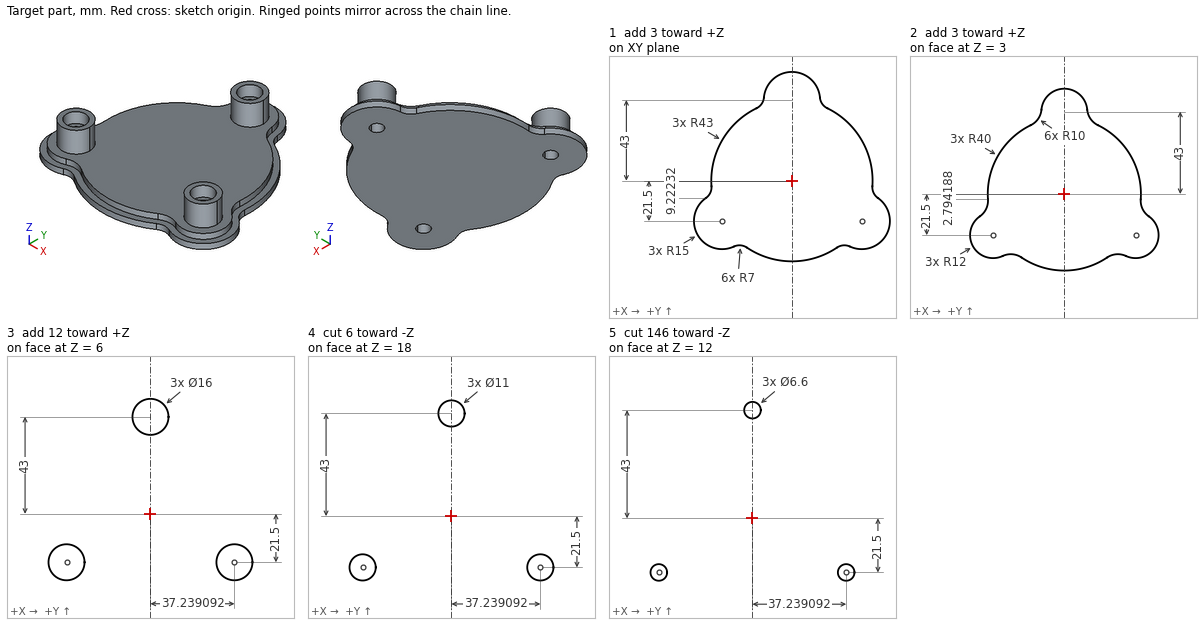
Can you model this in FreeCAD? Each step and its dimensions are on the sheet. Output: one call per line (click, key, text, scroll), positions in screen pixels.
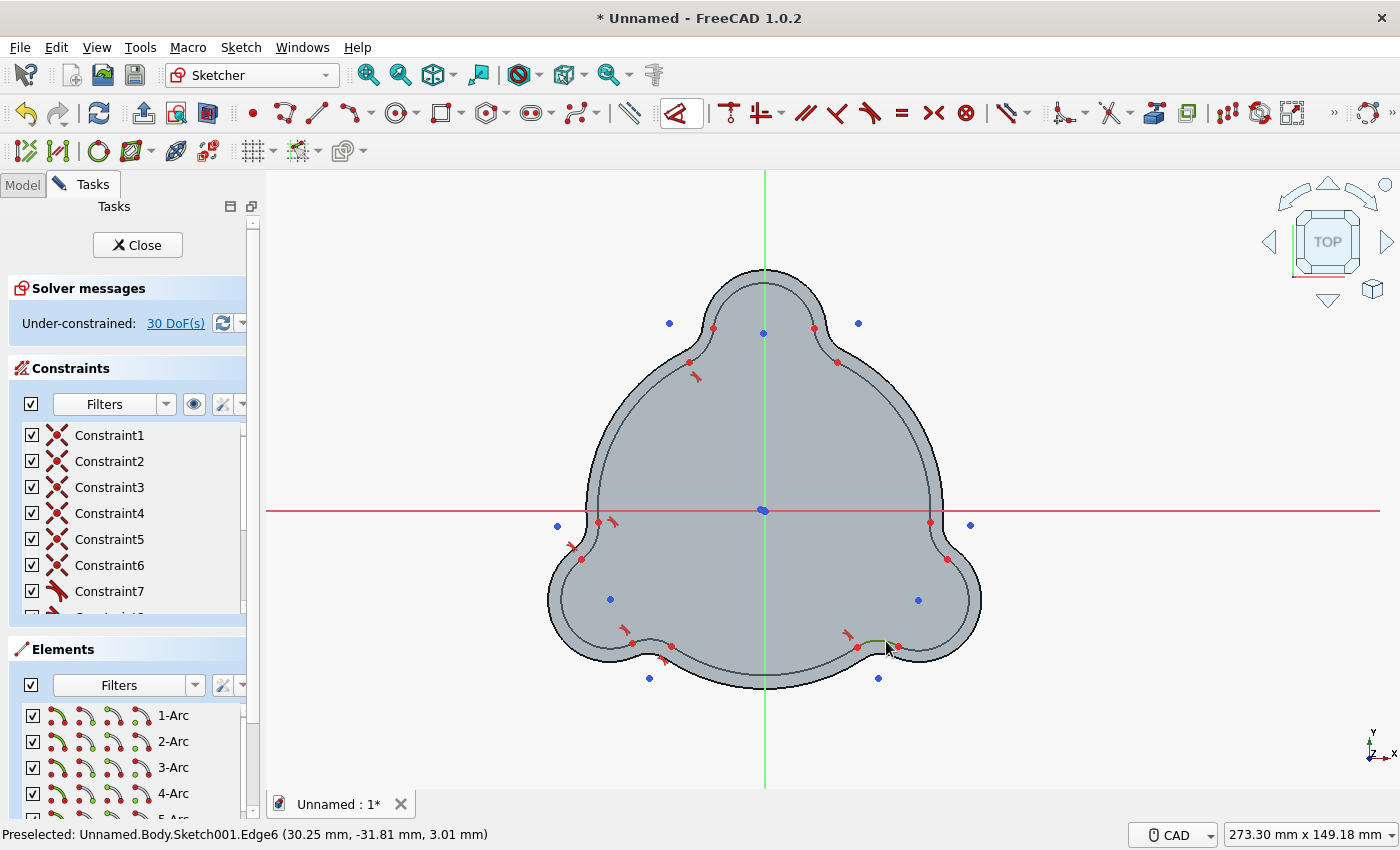
click(941, 645)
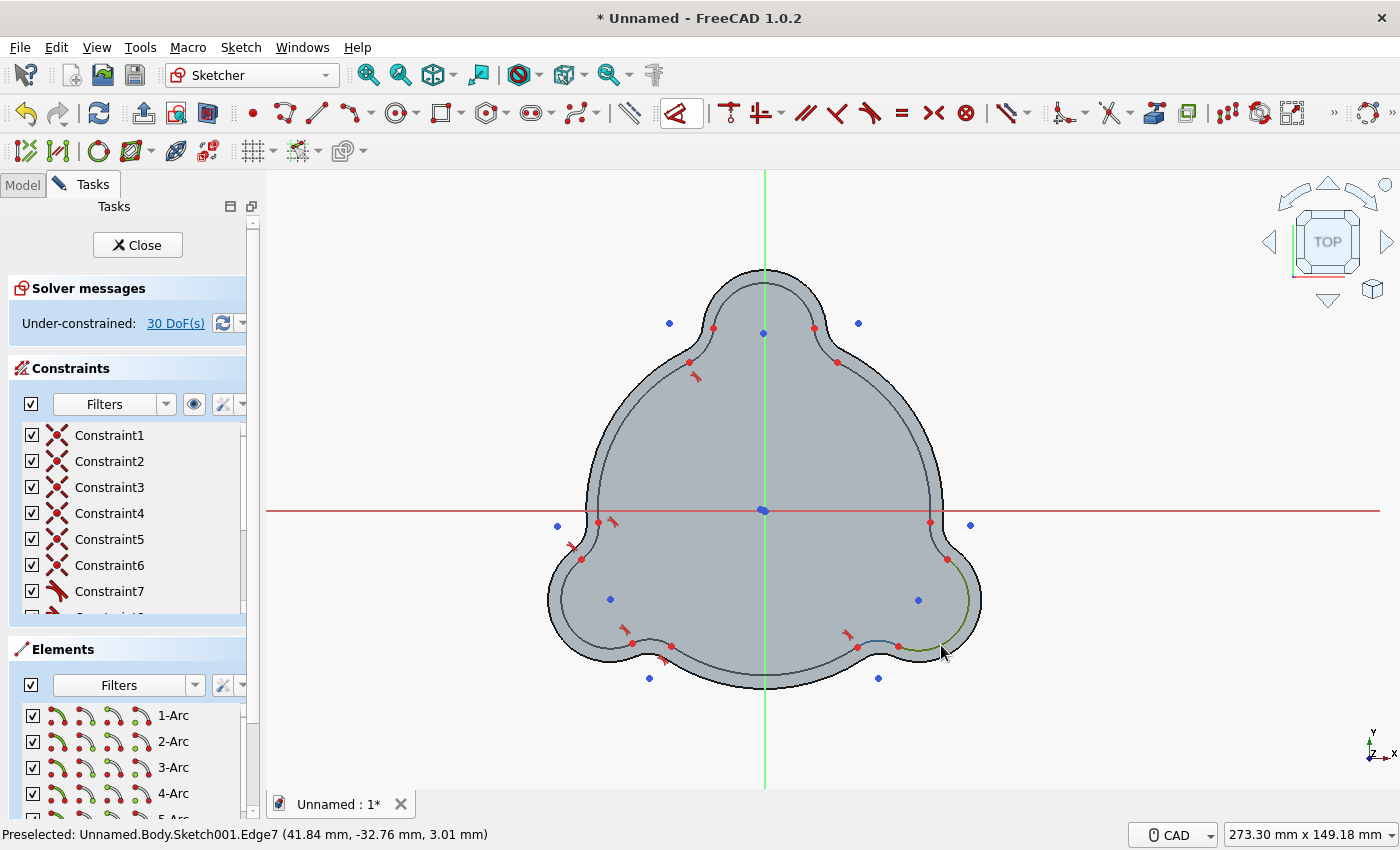
key(t)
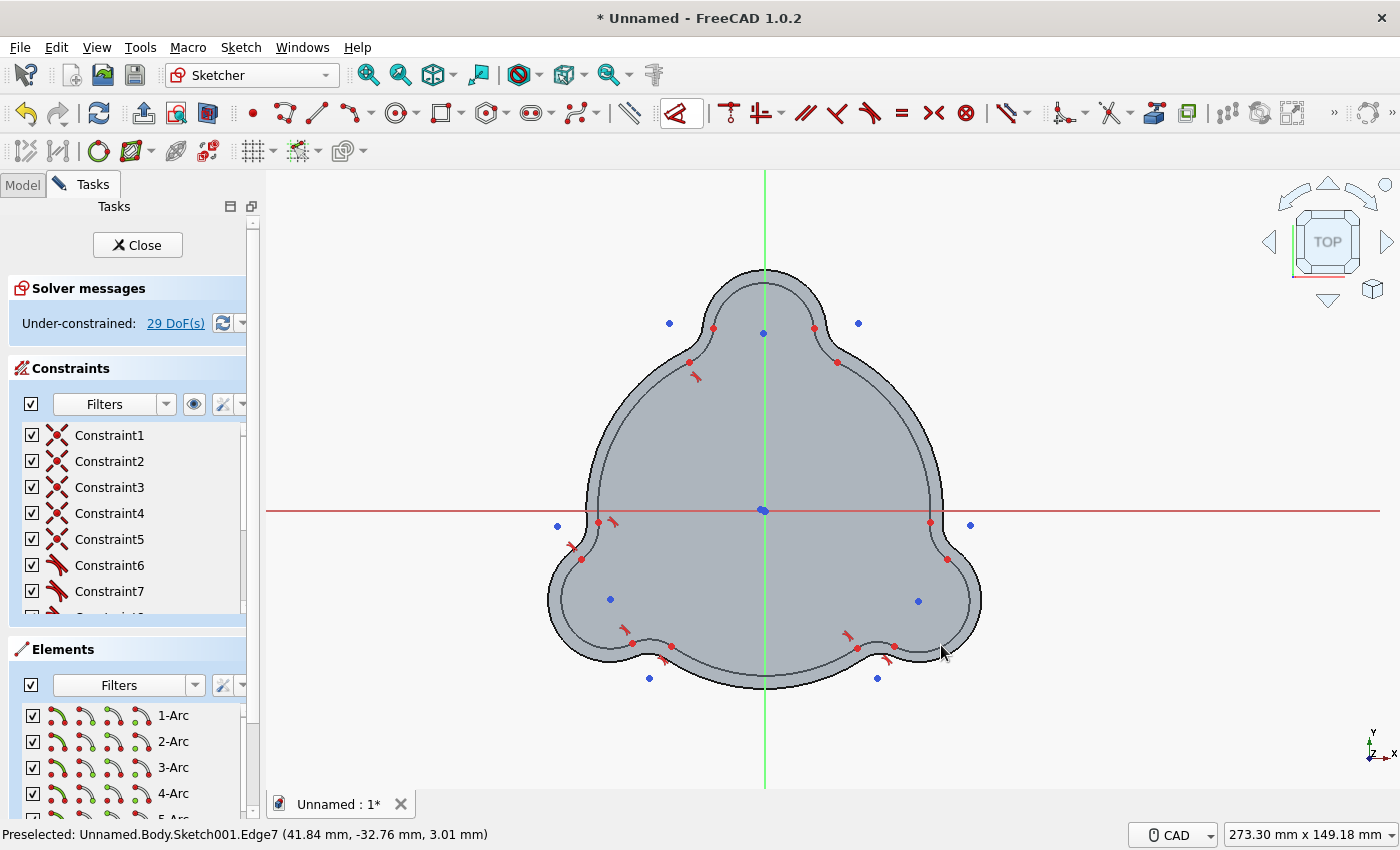
click(939, 648)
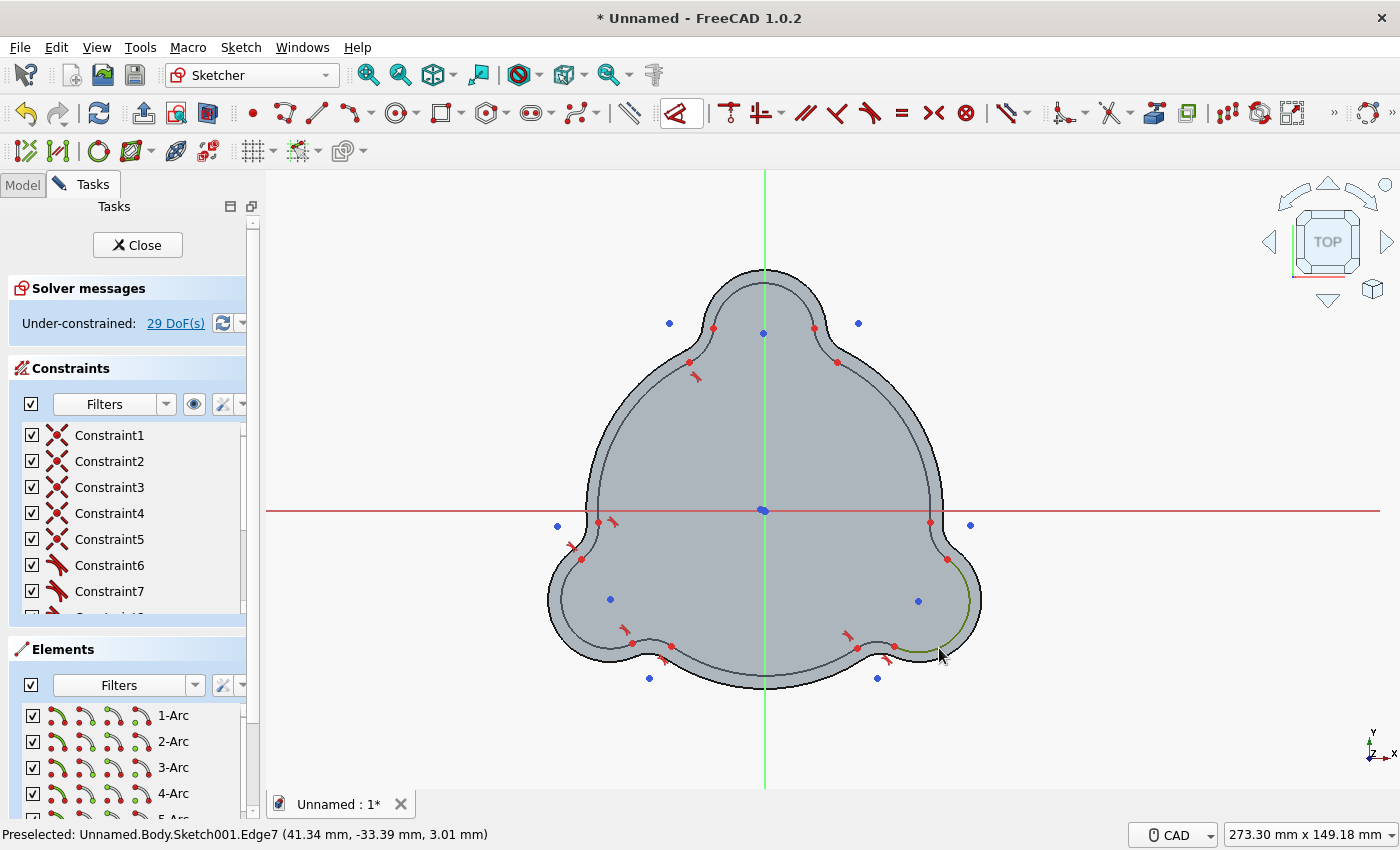
click(931, 535)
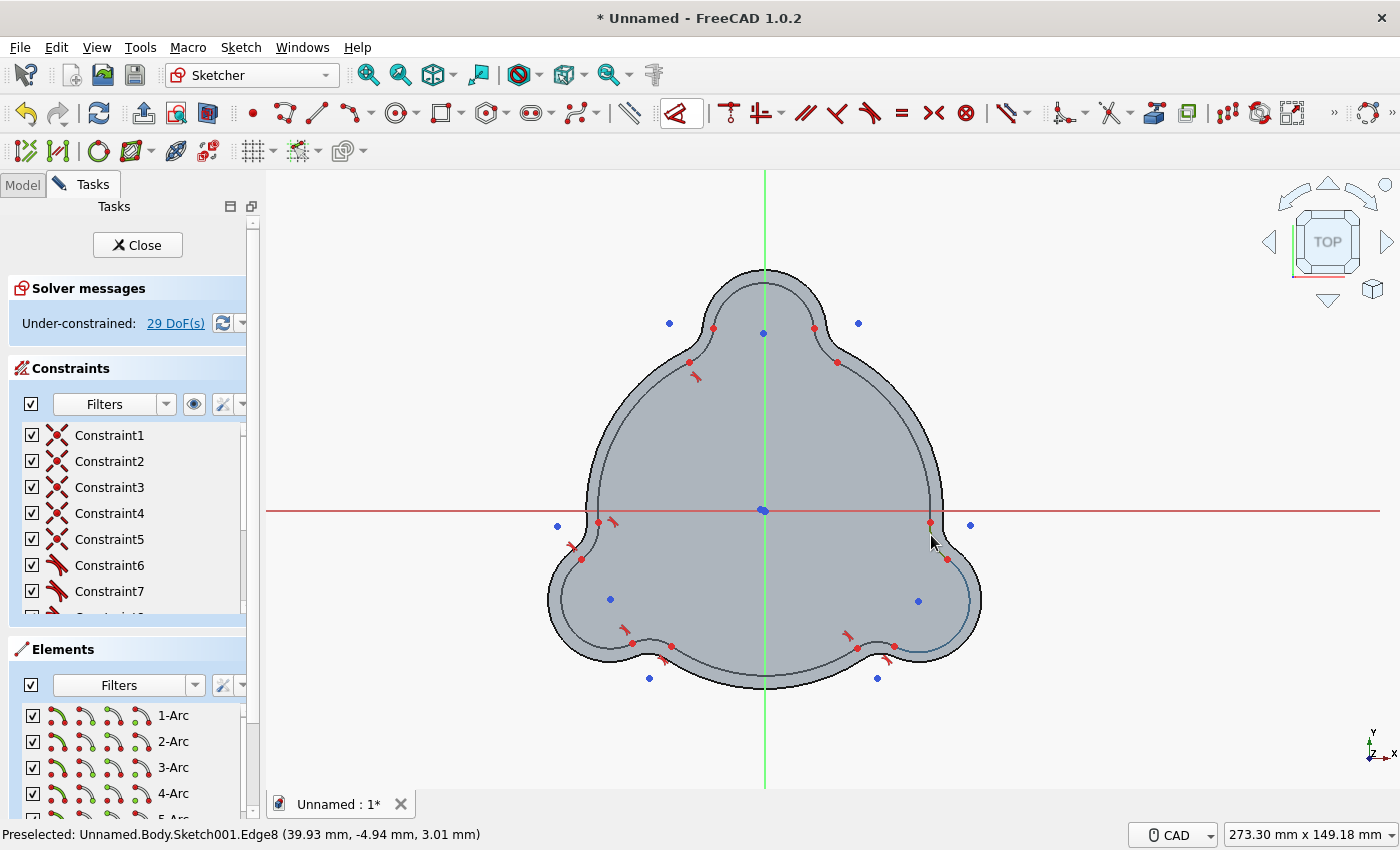
click(870, 114)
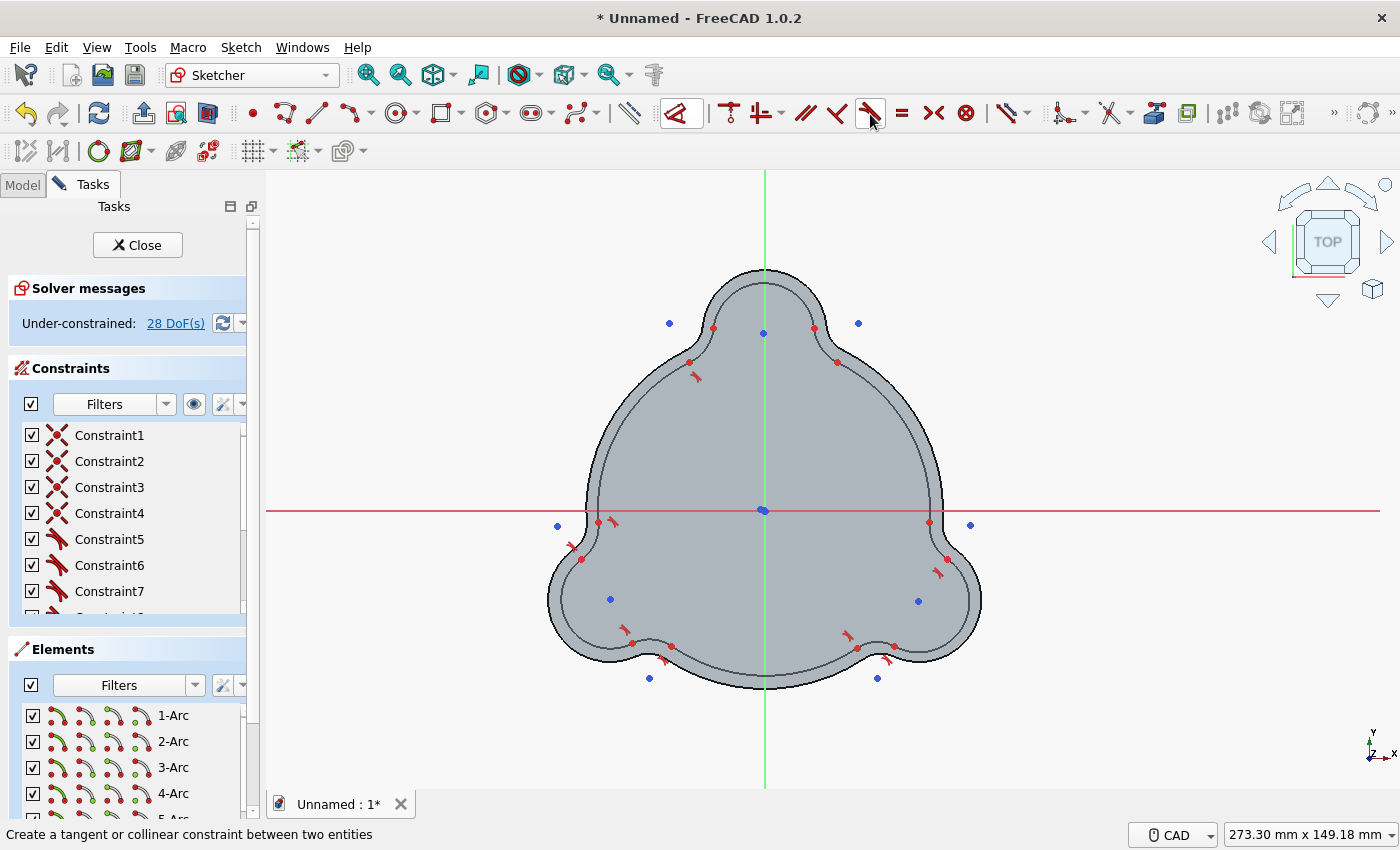
click(931, 535)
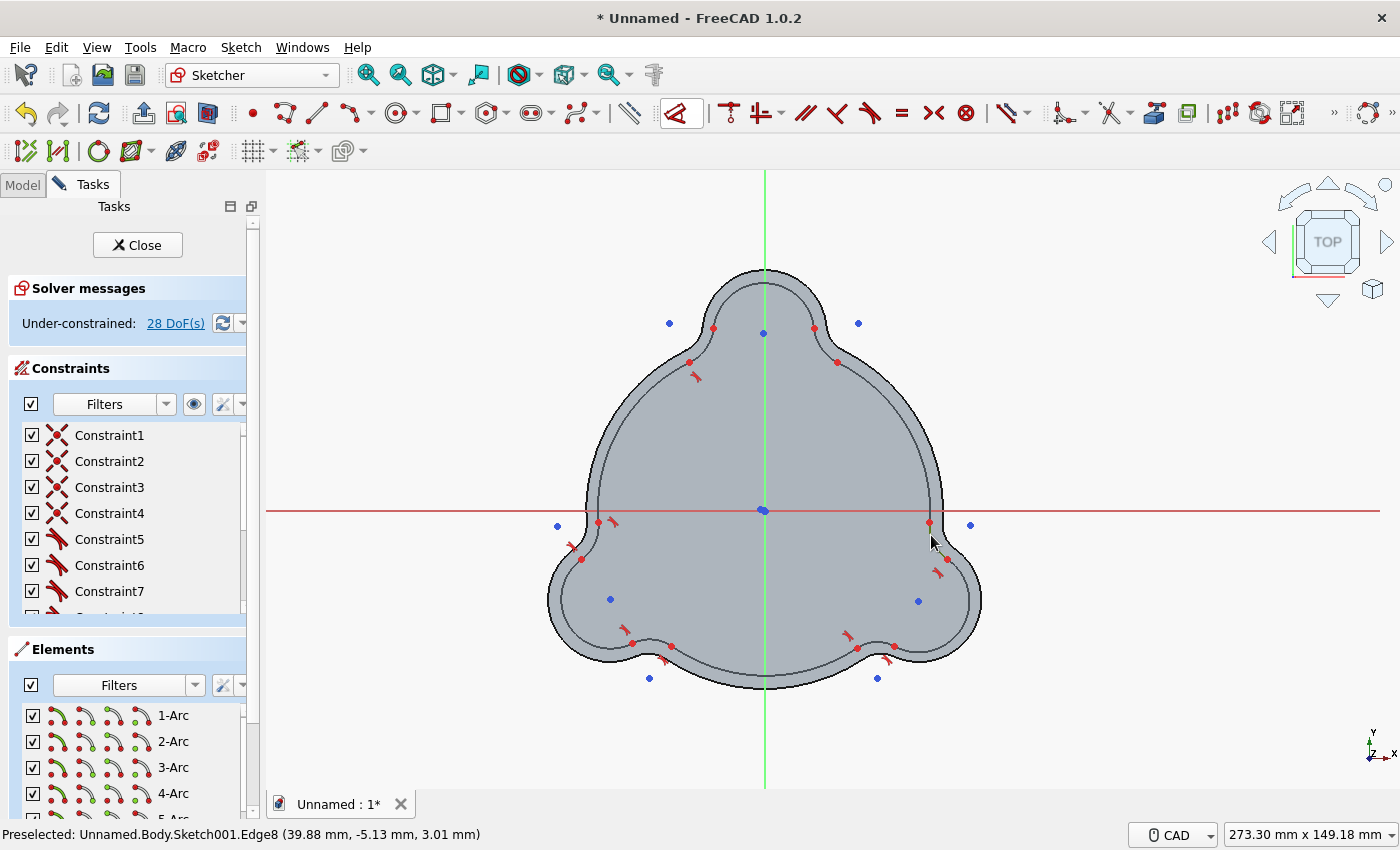
click(923, 464)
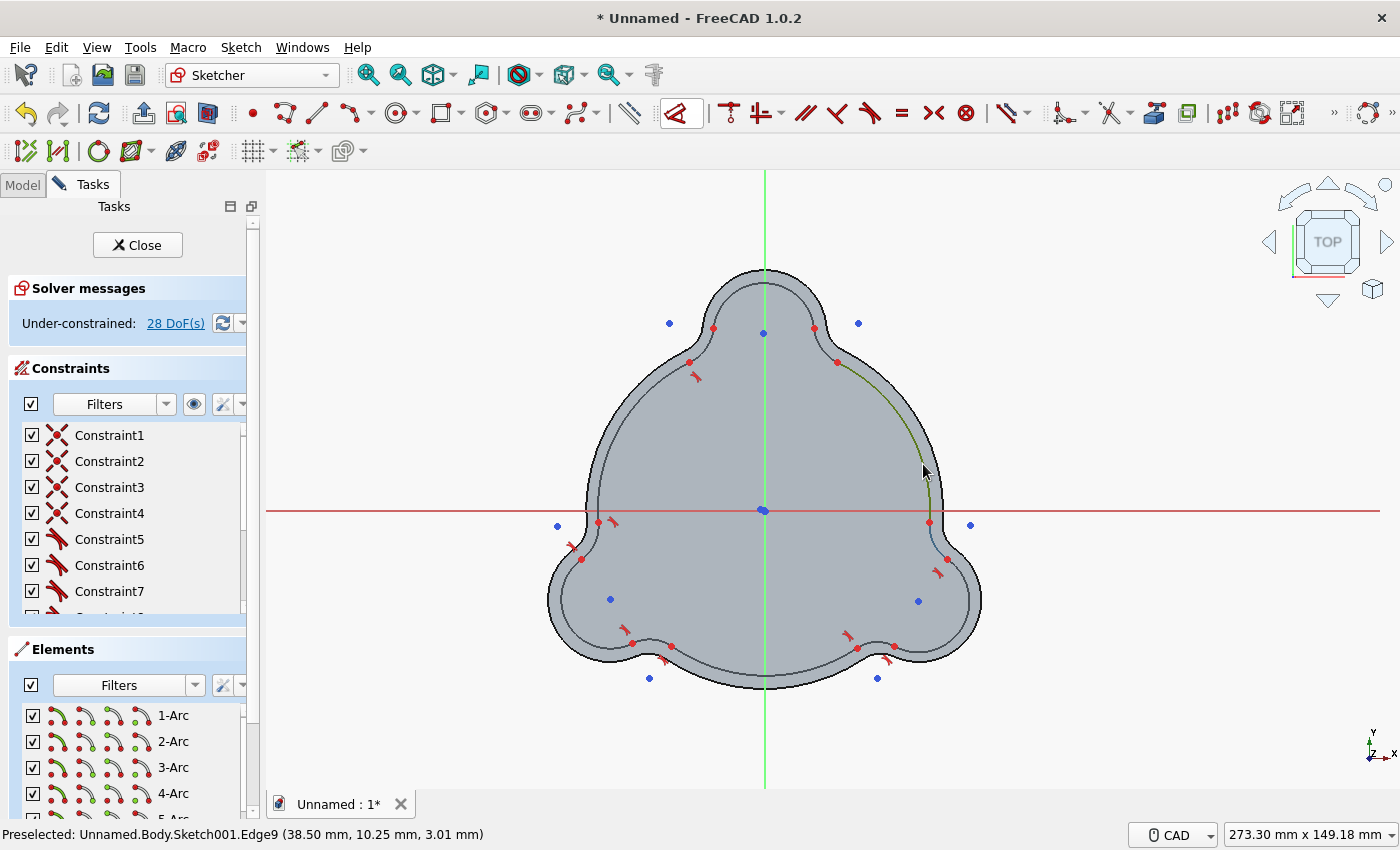
click(870, 114)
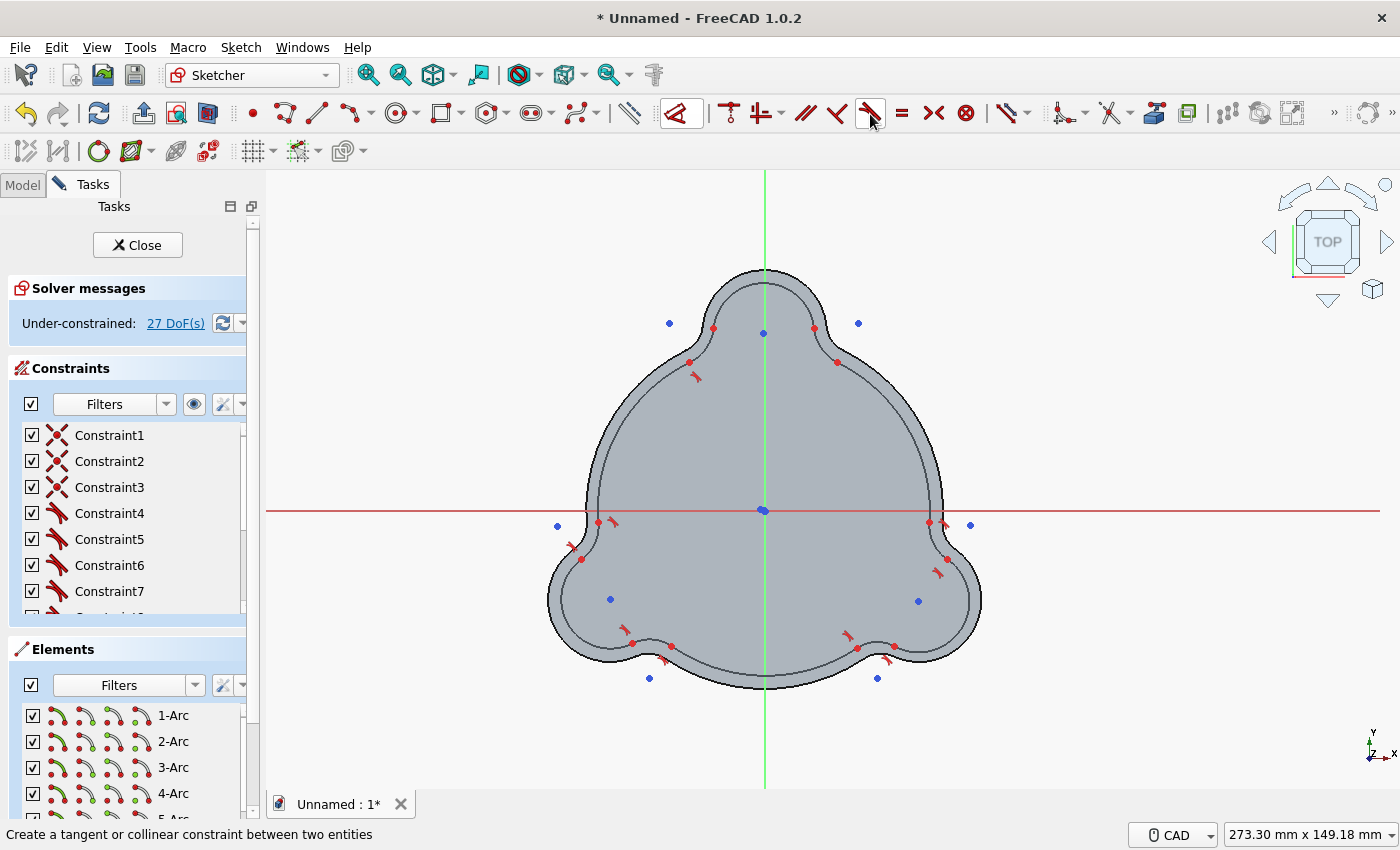
click(923, 464)